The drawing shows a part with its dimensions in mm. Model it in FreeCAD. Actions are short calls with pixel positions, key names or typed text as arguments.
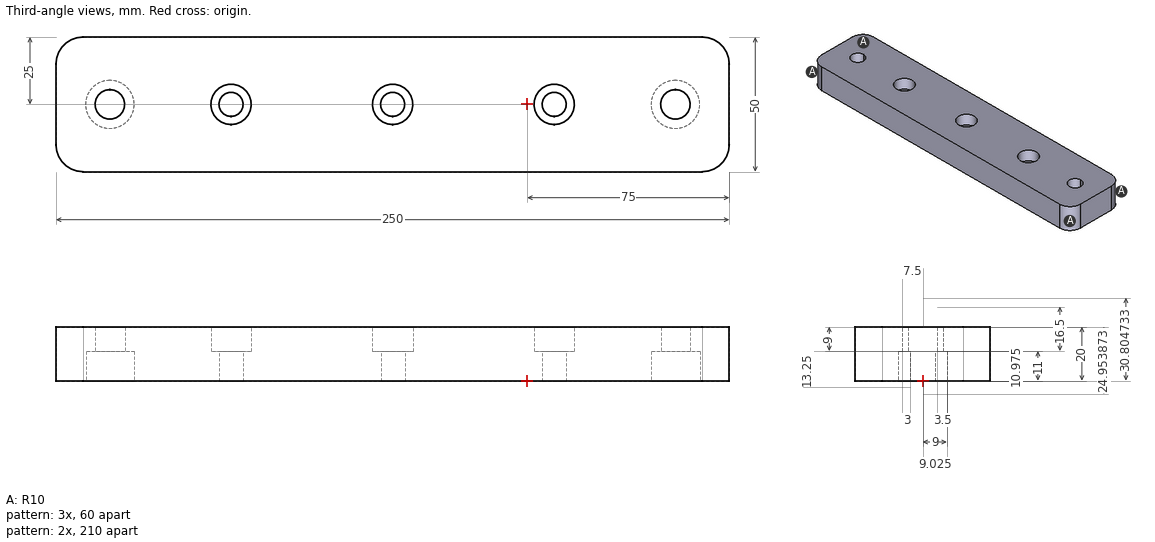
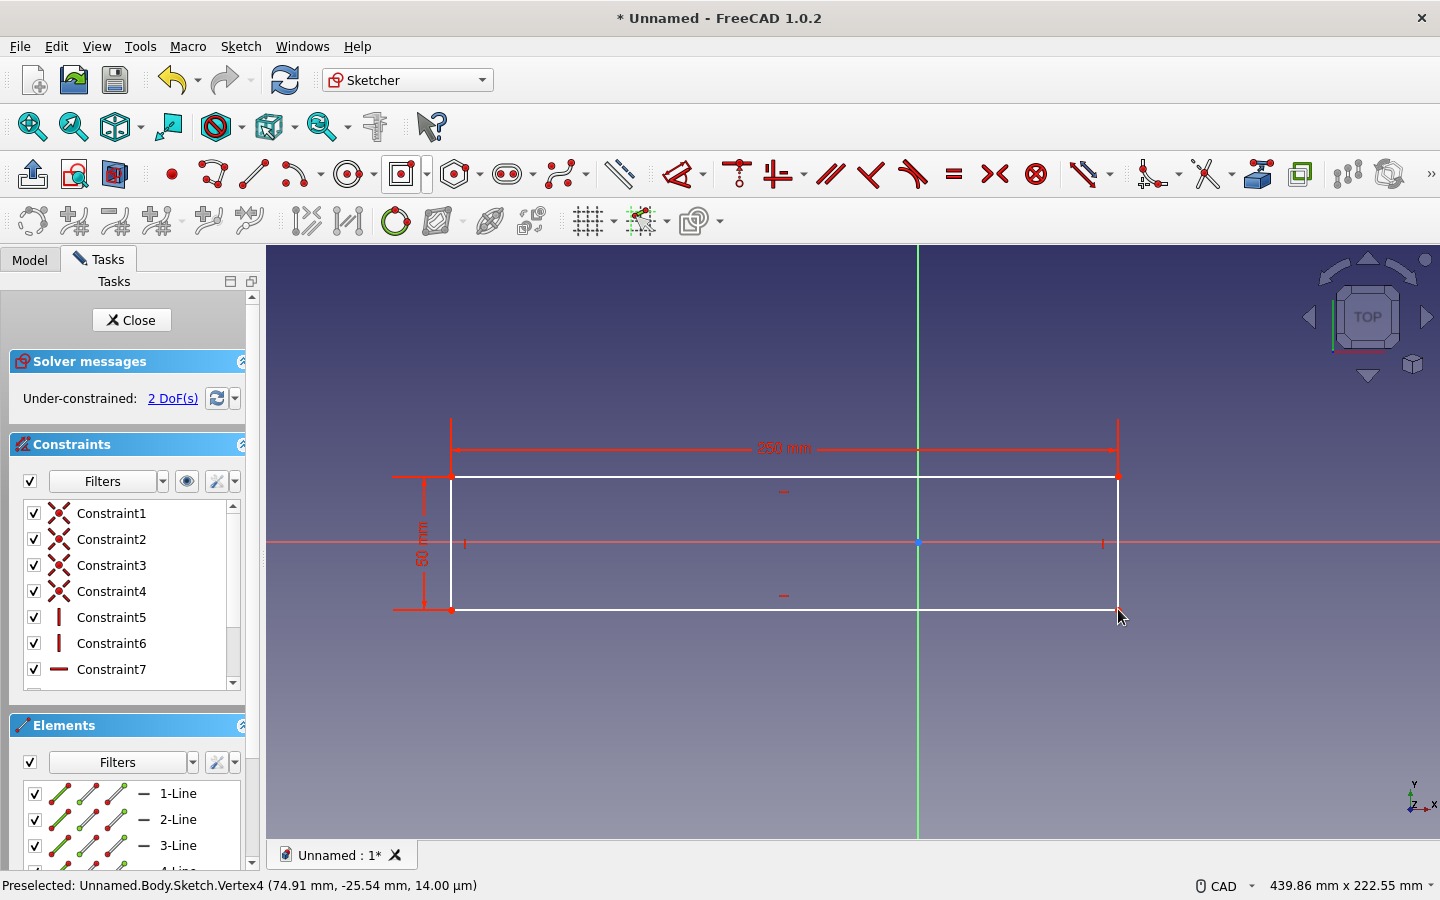
click(451, 477)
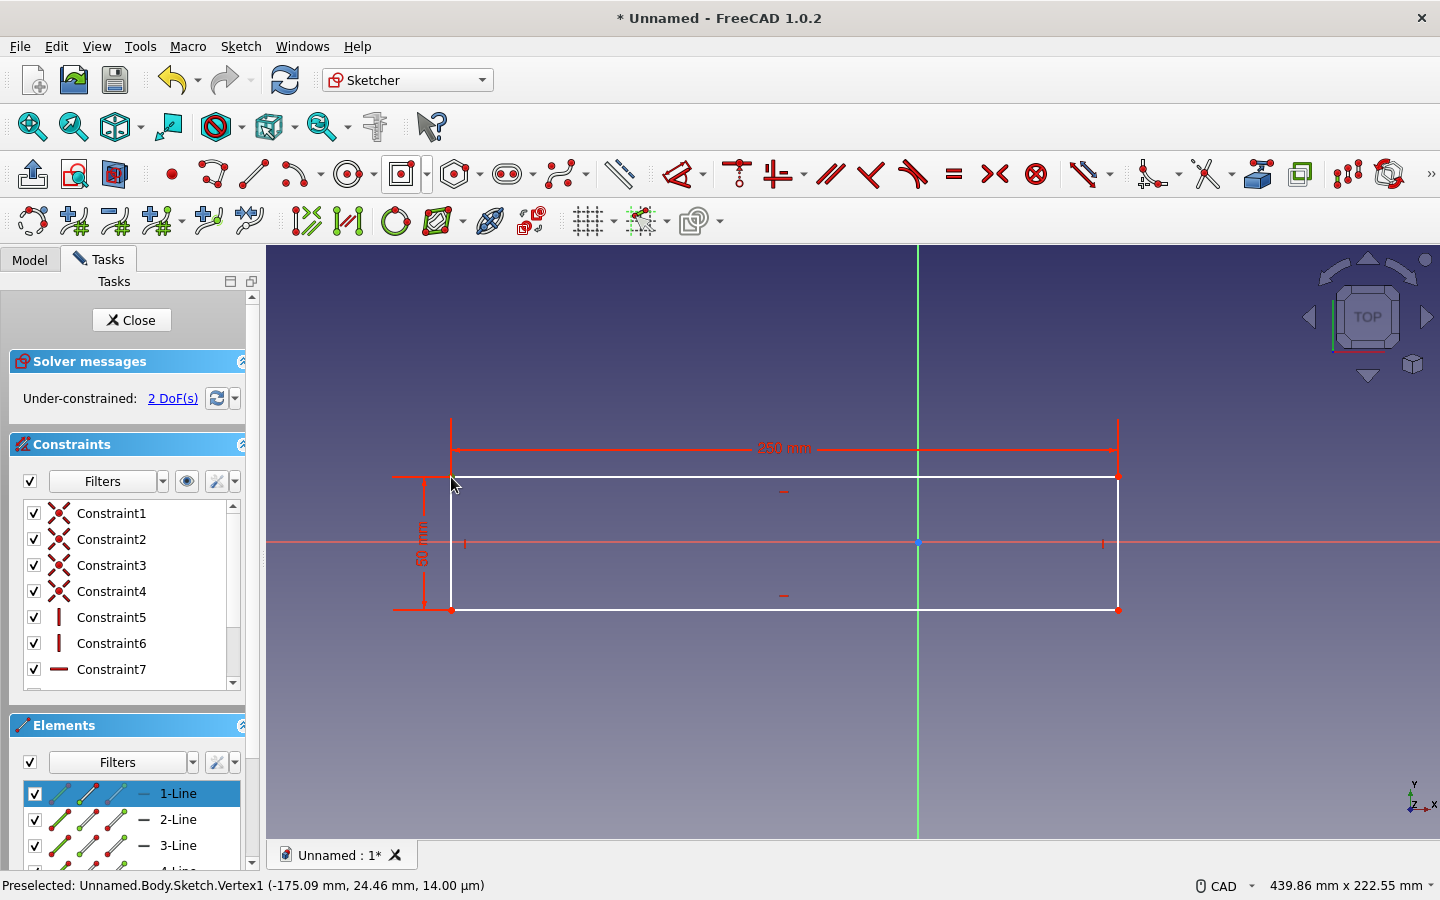
key(i)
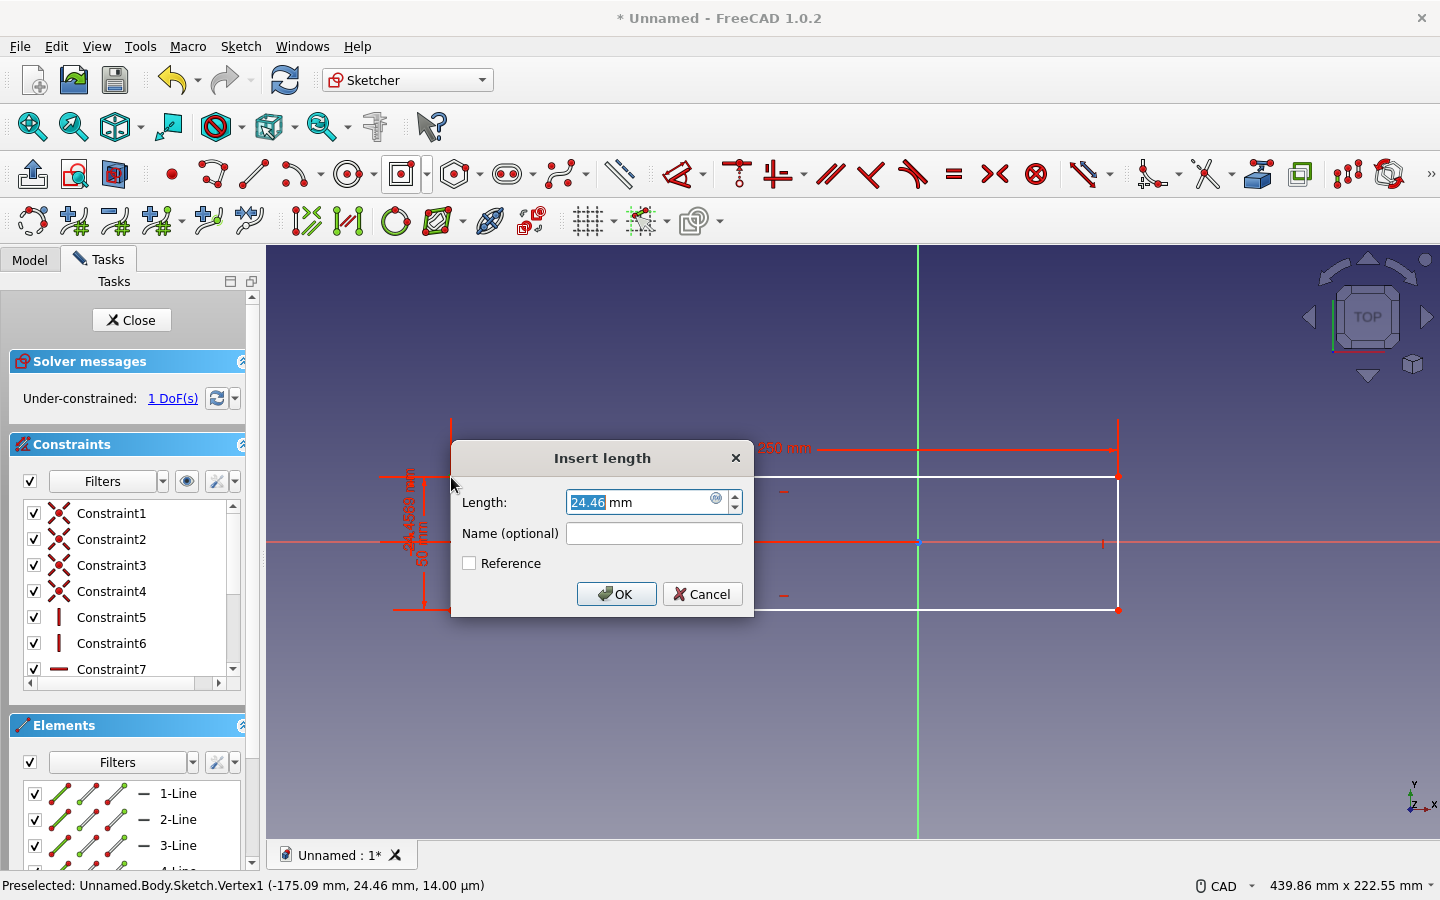
text(25)
key(Return)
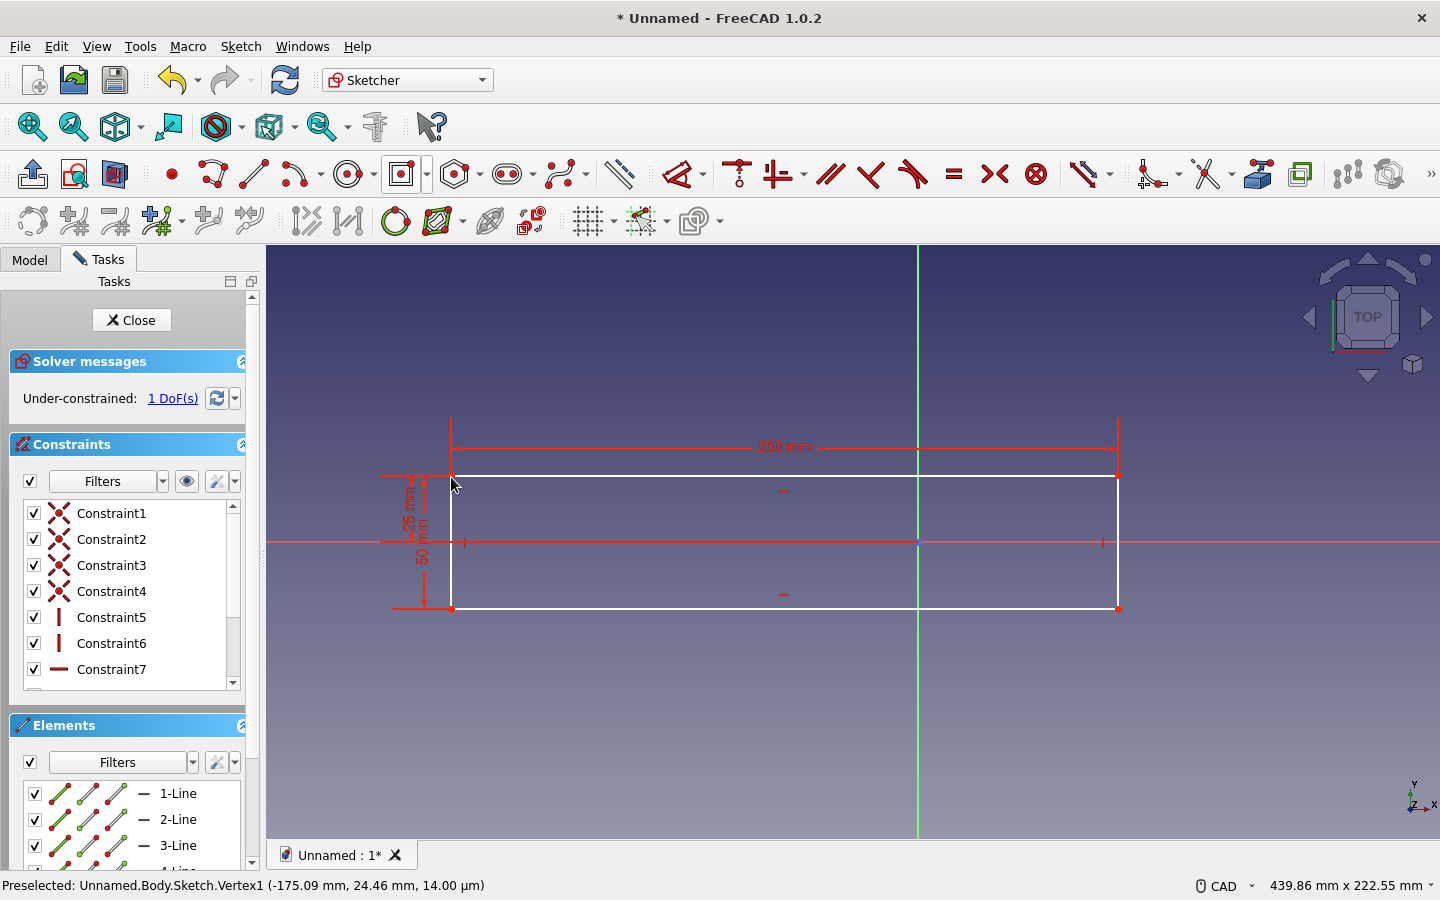
click(1118, 609)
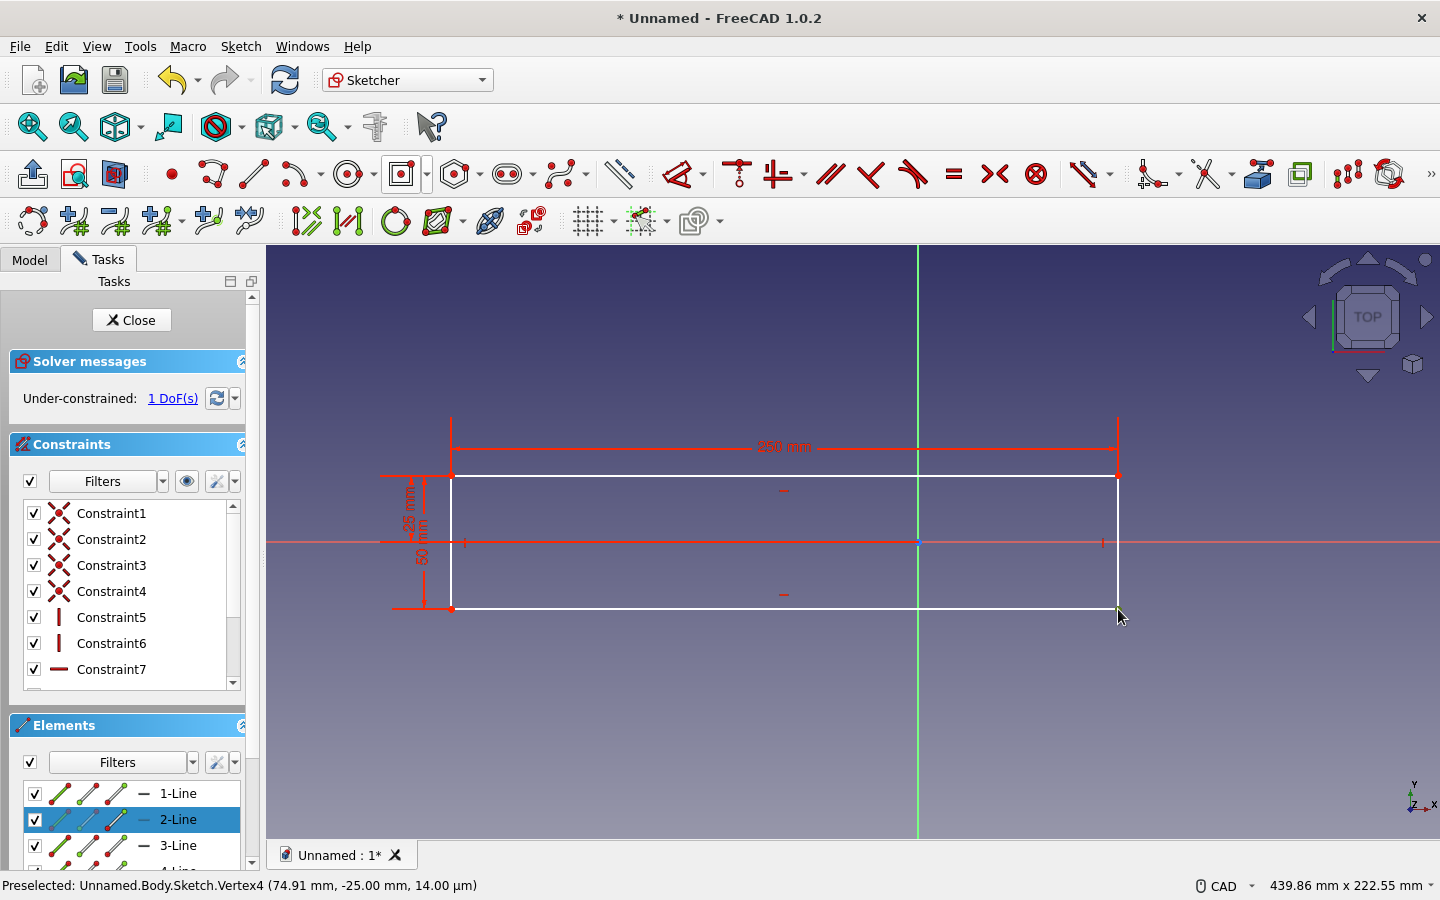
key(l)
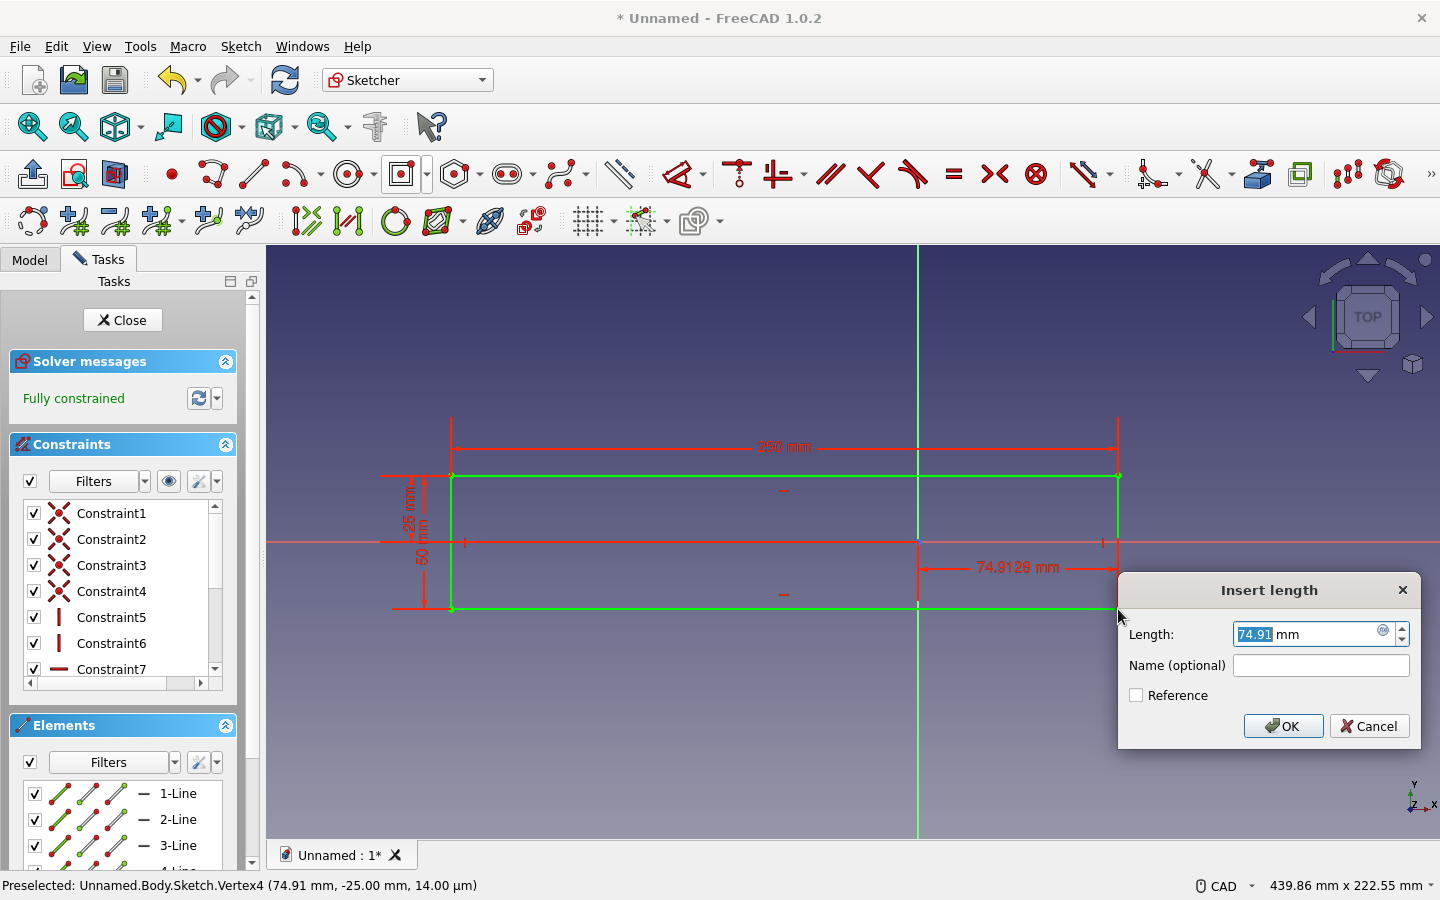
text(75)
key(Return)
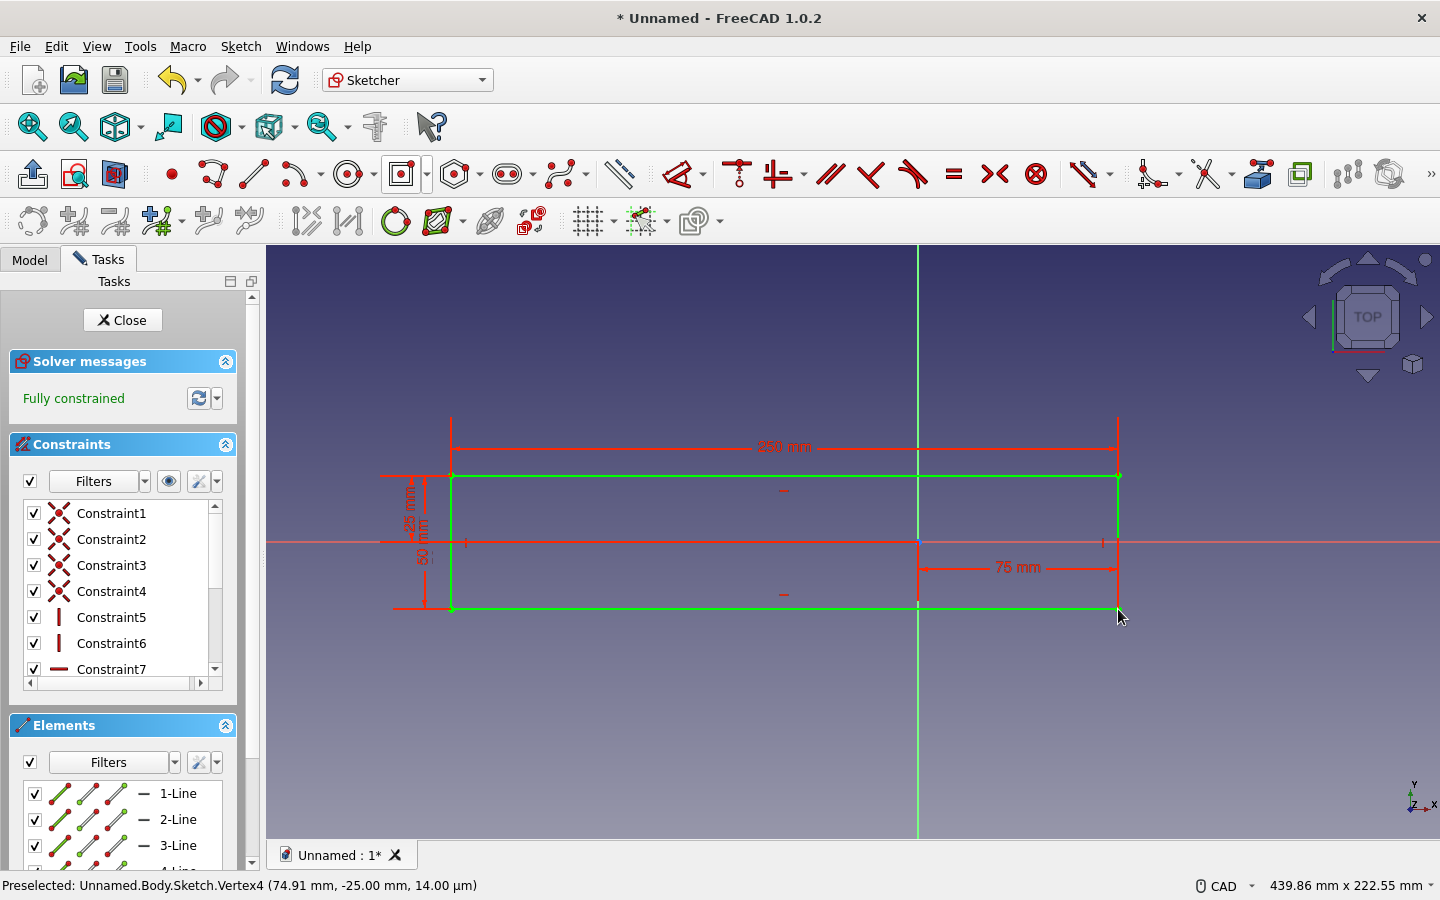
click(123, 320)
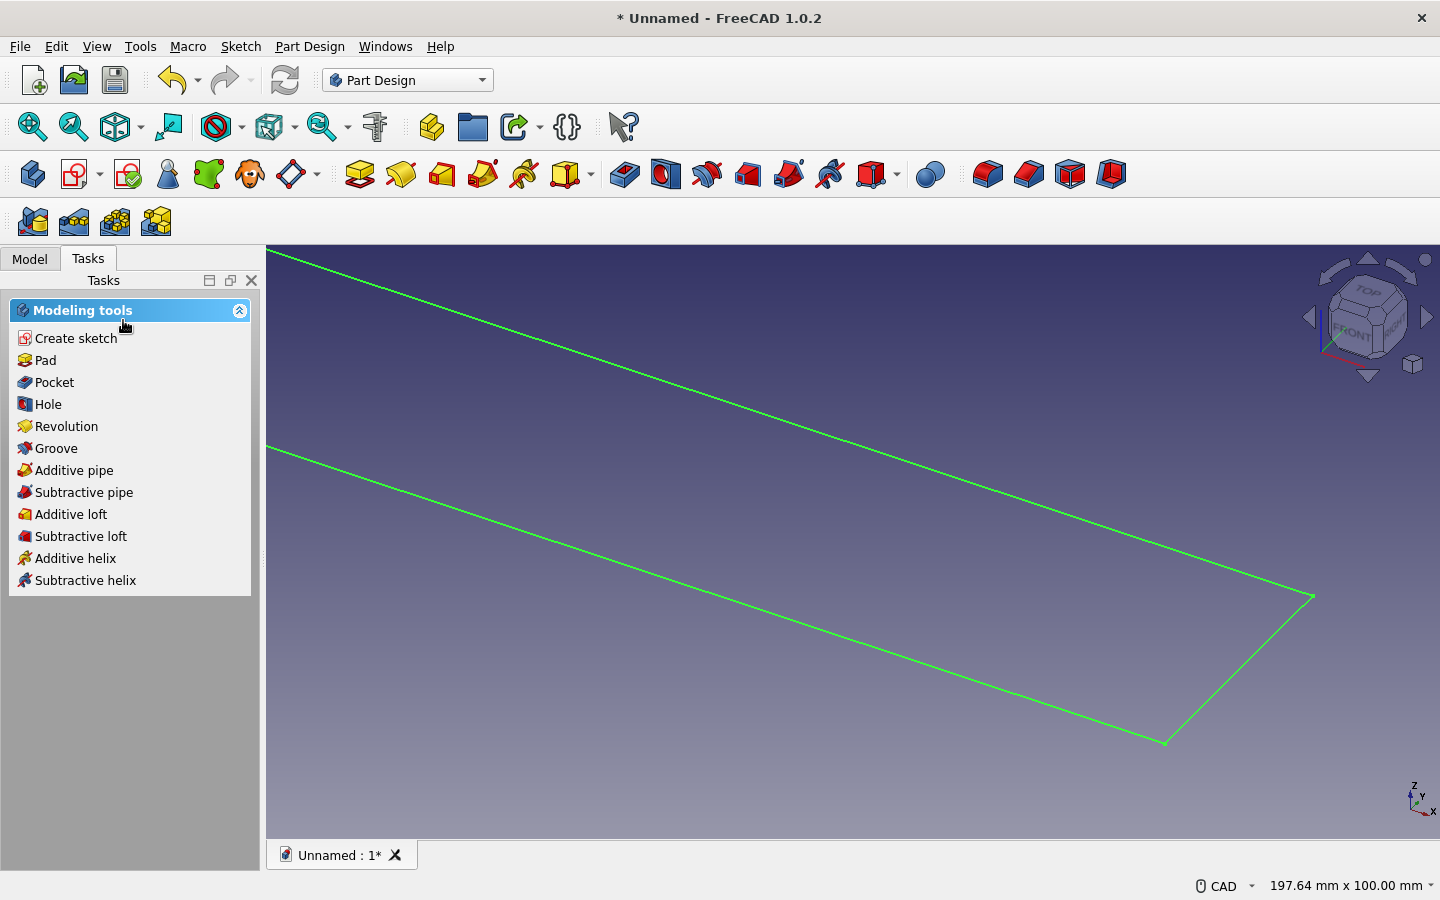
click(360, 174)